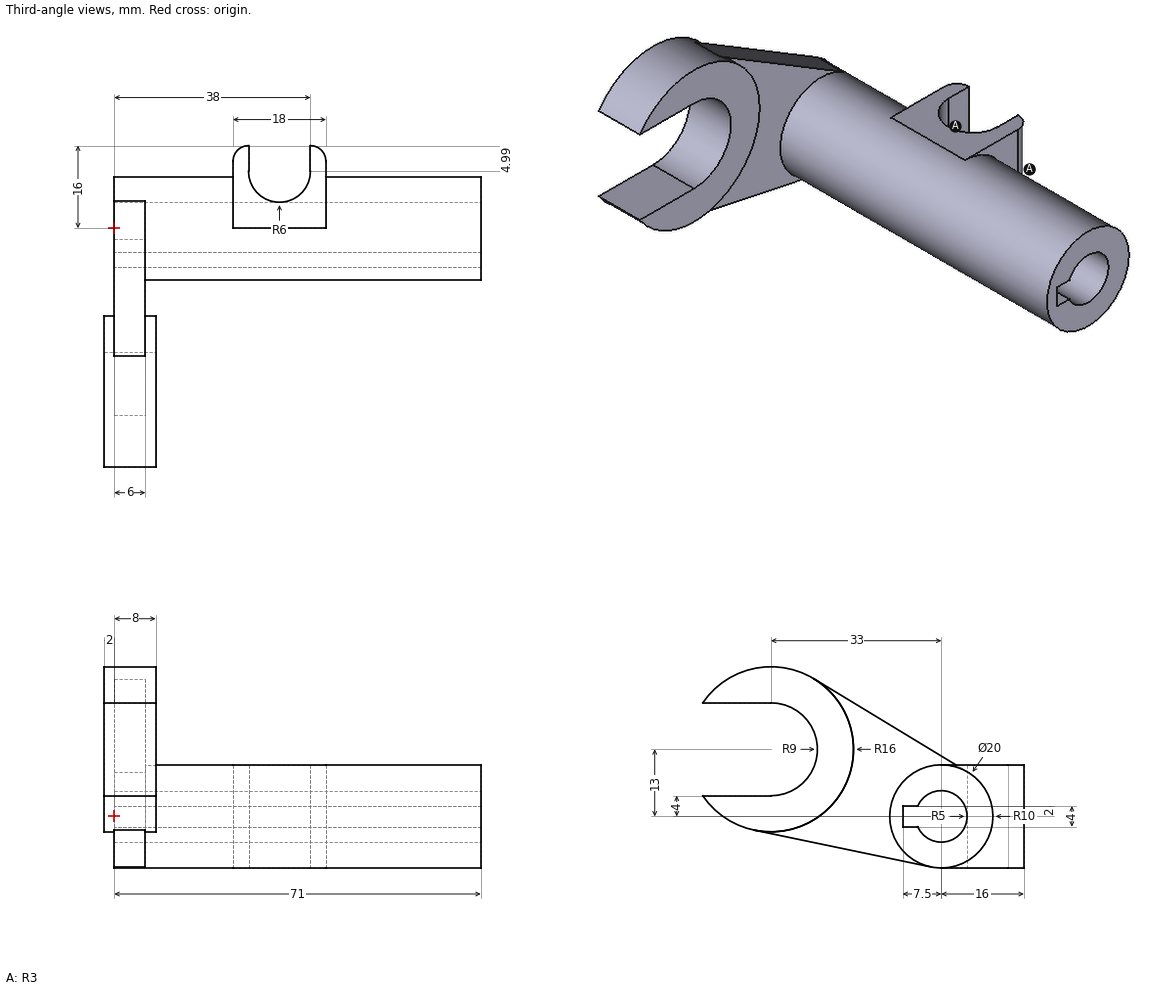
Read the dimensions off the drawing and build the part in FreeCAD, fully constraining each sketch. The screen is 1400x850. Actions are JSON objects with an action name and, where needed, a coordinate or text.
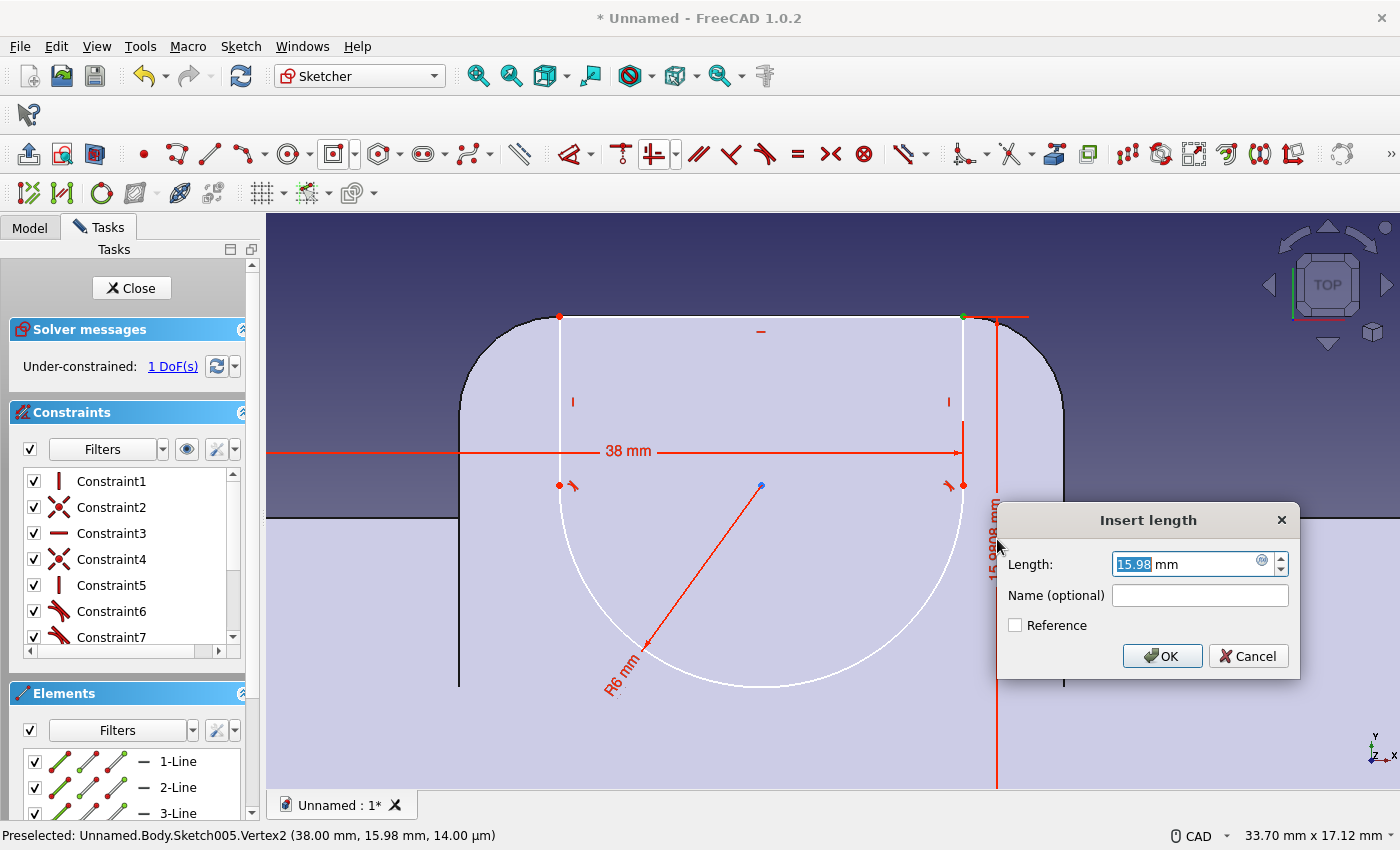
{"action": "type", "text": "16"}
{"action": "key", "text": "Return"}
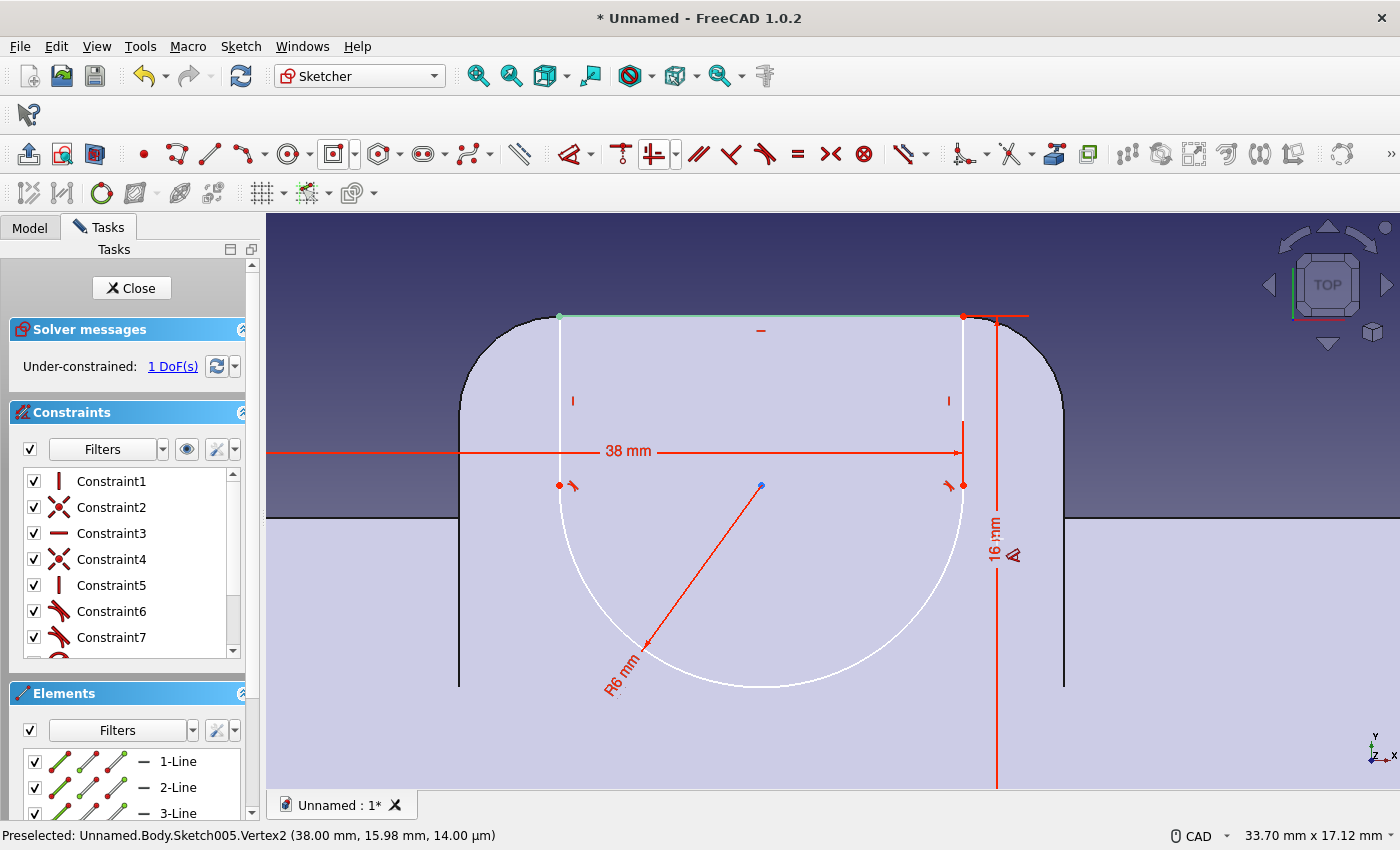
{"action": "left_click", "coordinate": [963, 435]}
{"action": "left_click", "coordinate": [997, 401]}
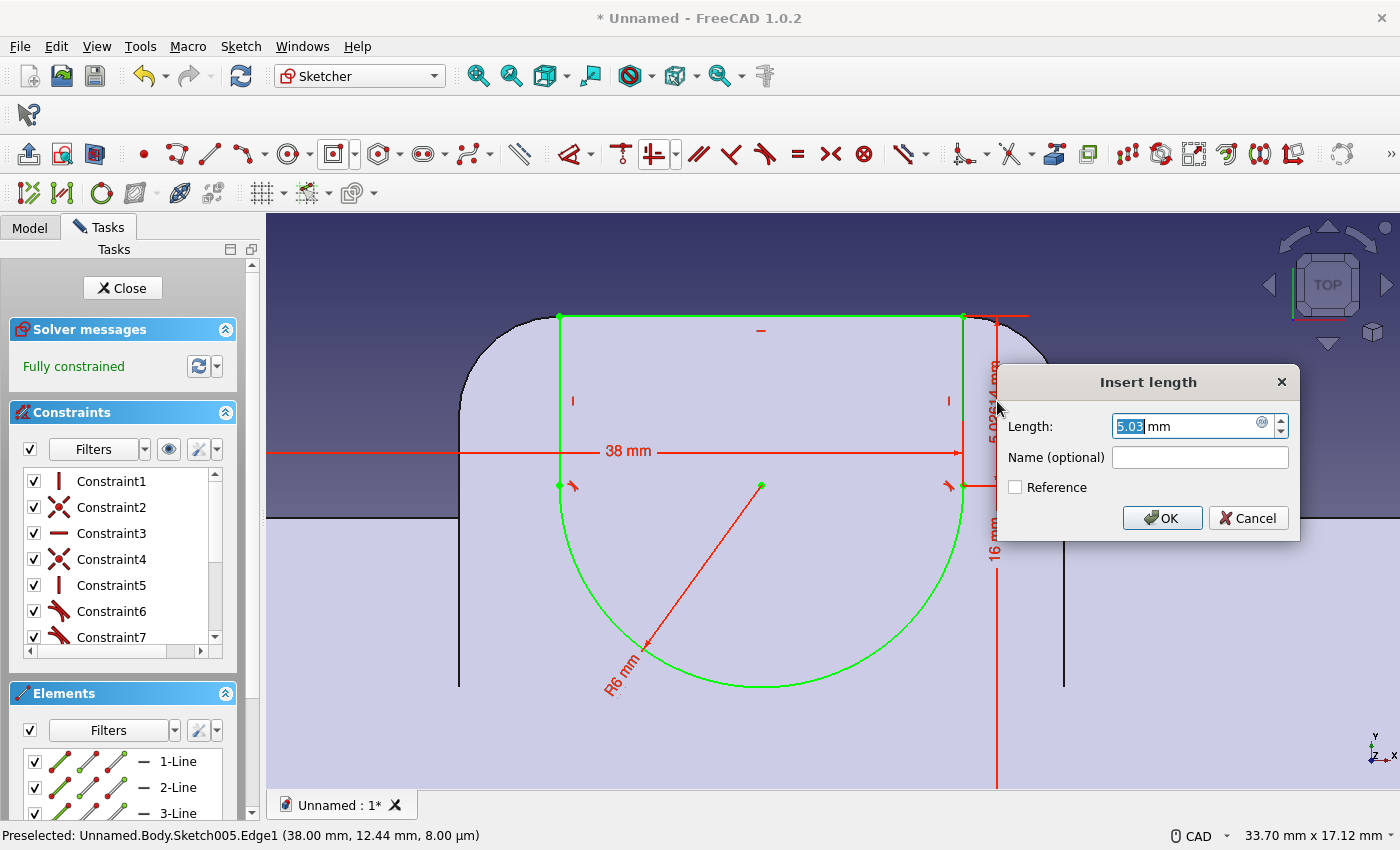
{"action": "type", "text": "4.99"}
{"action": "key", "text": "Return"}
{"action": "key", "text": "Escape"}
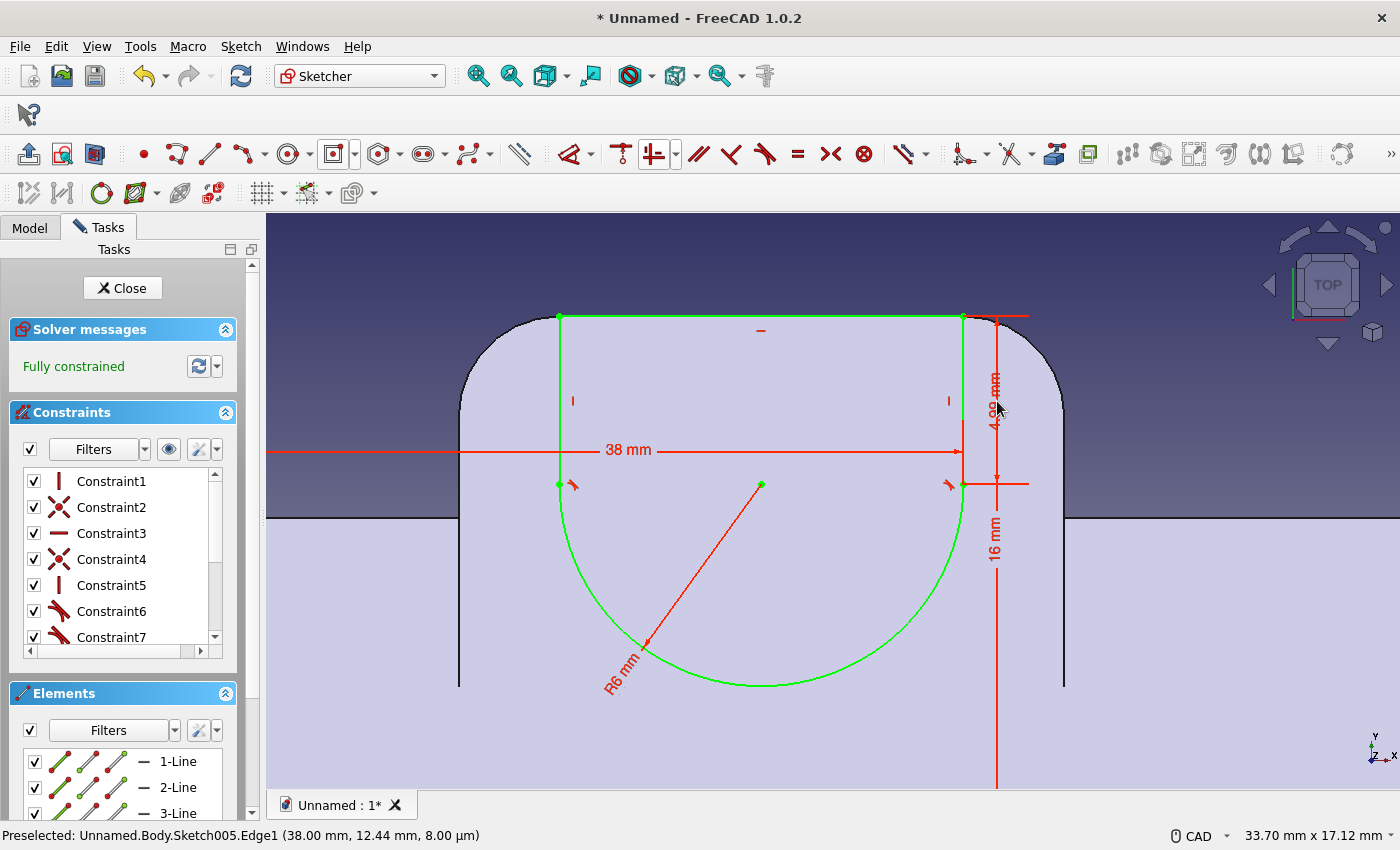
{"action": "left_click", "coordinate": [123, 288]}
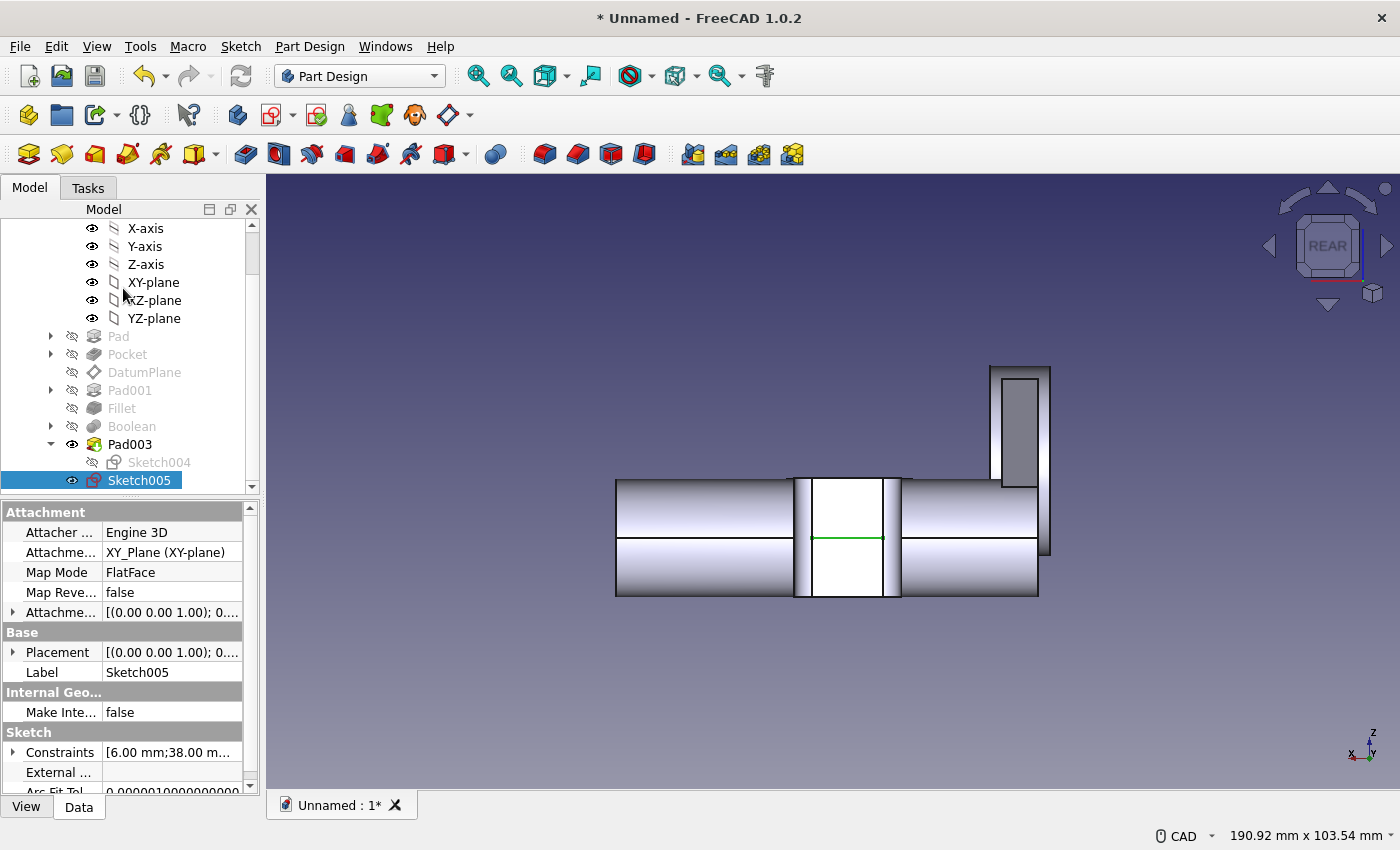
{"action": "left_click", "coordinate": [246, 154]}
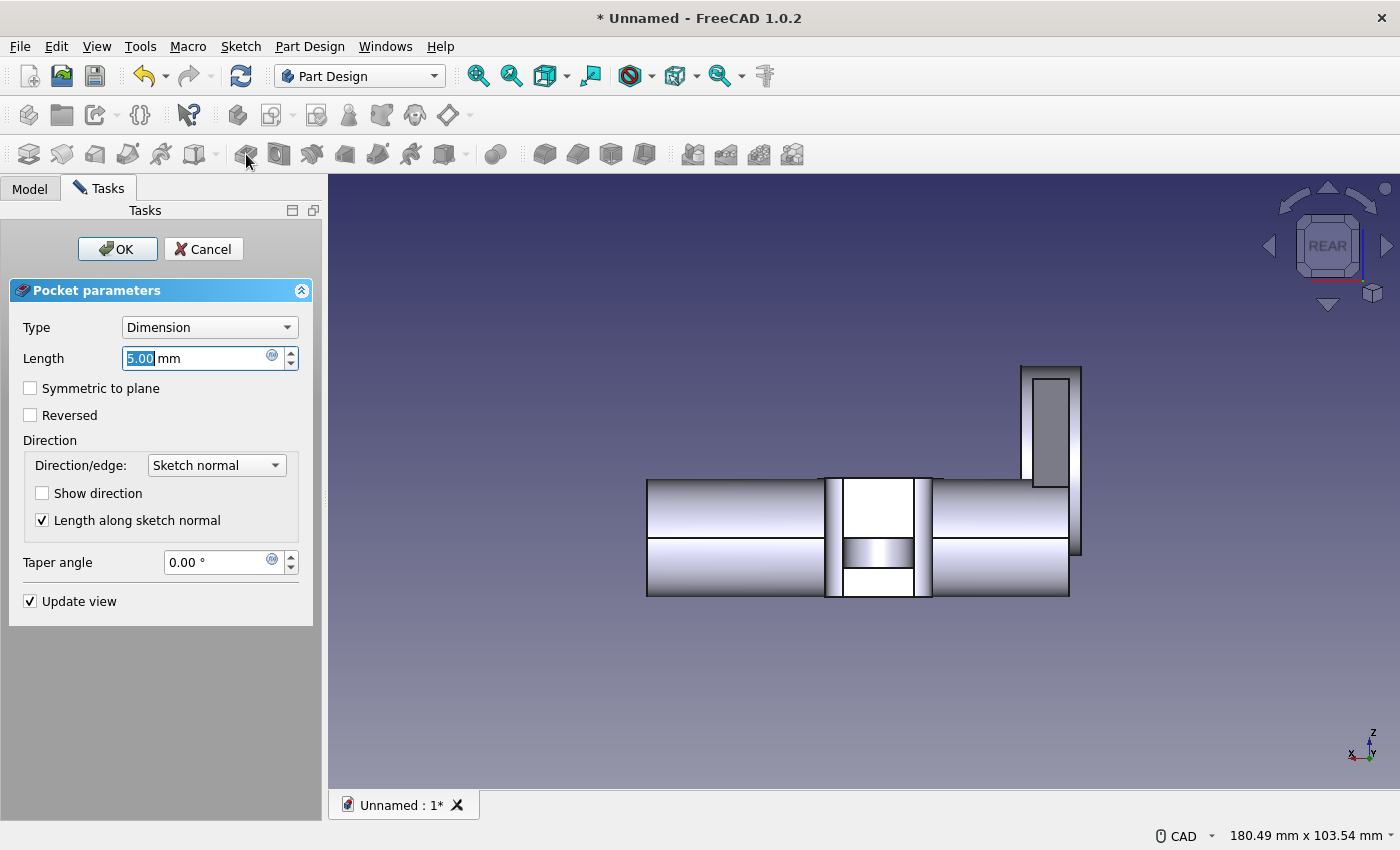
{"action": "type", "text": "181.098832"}
{"action": "key", "text": "Tab"}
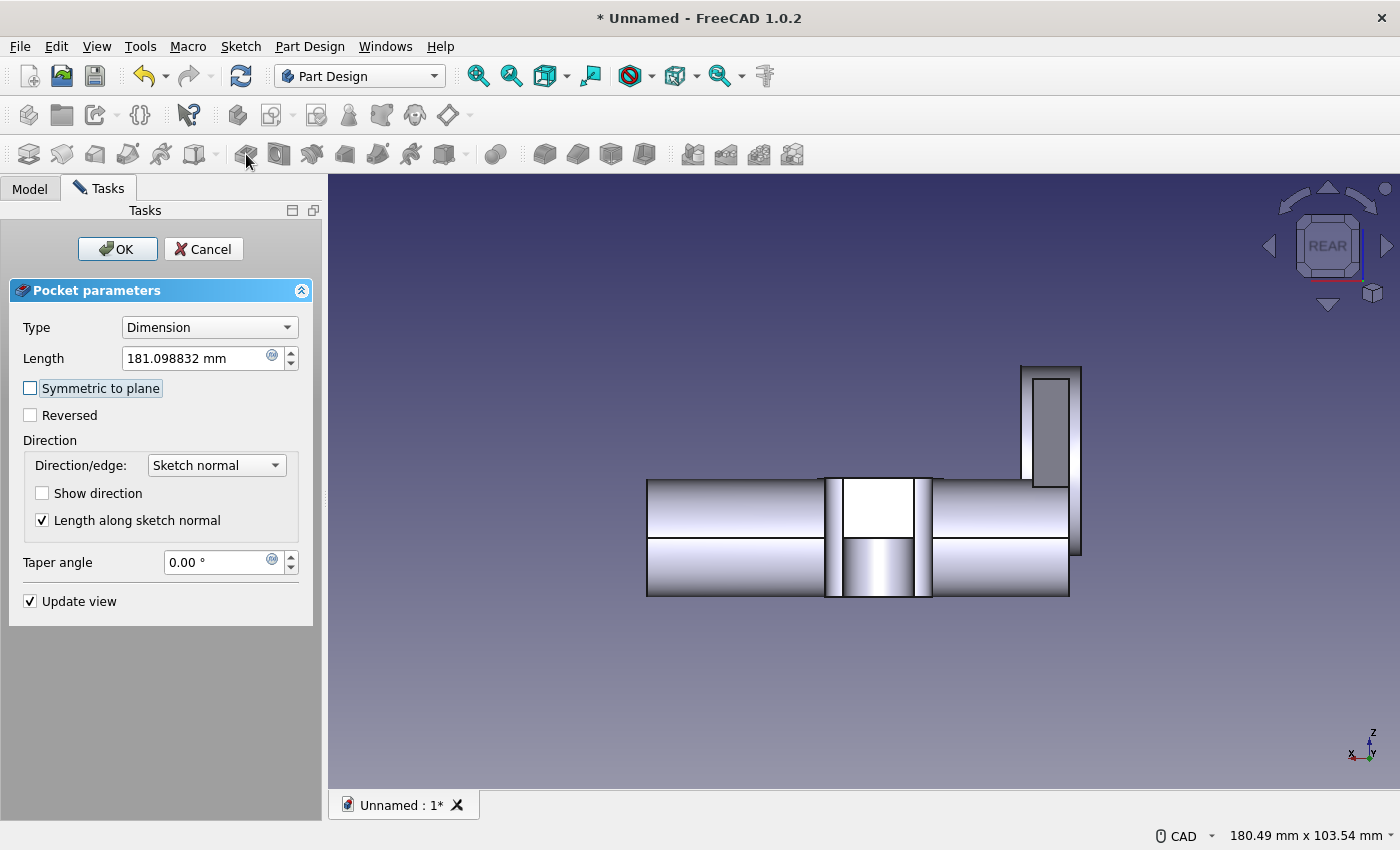
{"action": "left_click", "coordinate": [31, 388]}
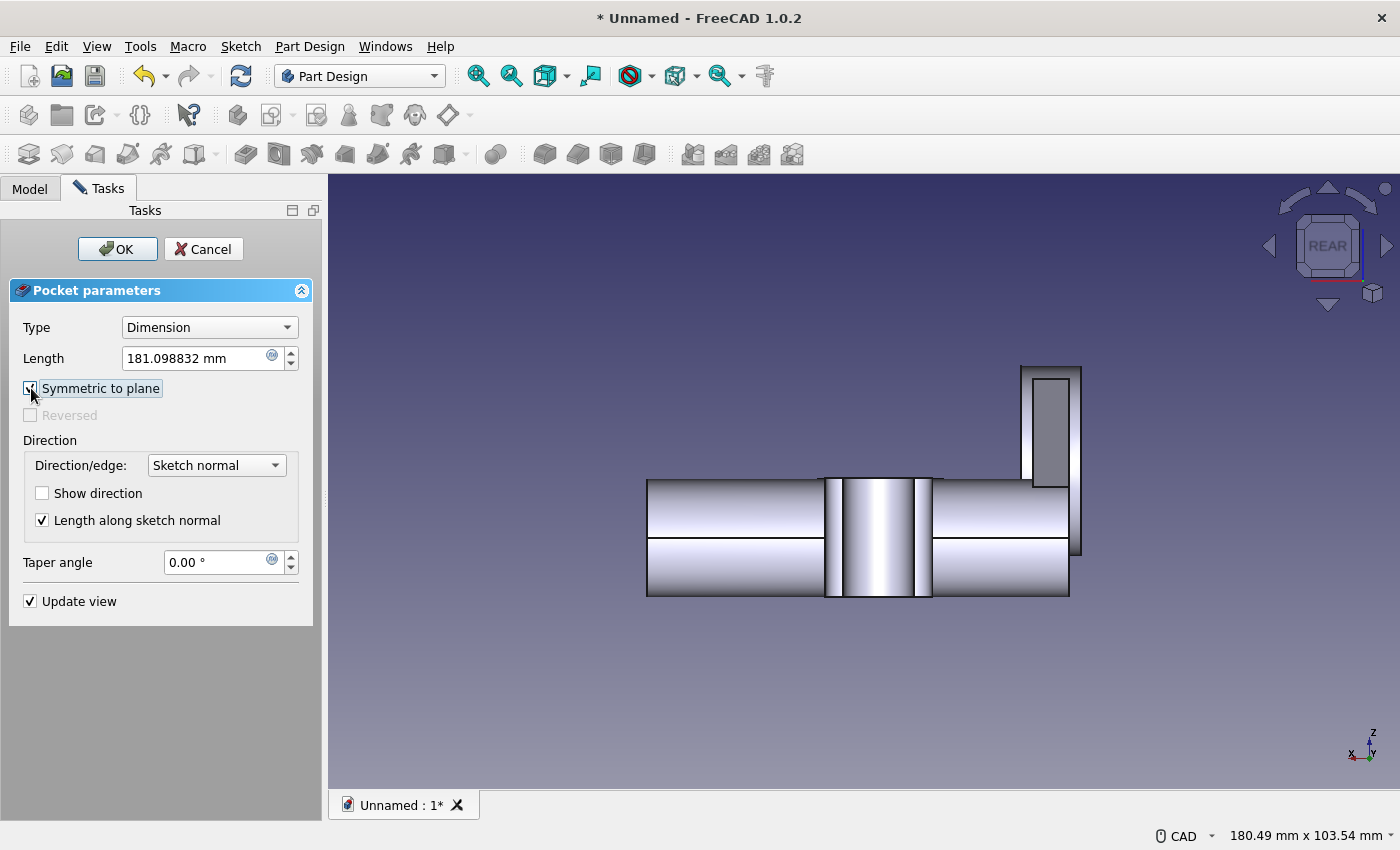
{"action": "left_click", "coordinate": [118, 249]}